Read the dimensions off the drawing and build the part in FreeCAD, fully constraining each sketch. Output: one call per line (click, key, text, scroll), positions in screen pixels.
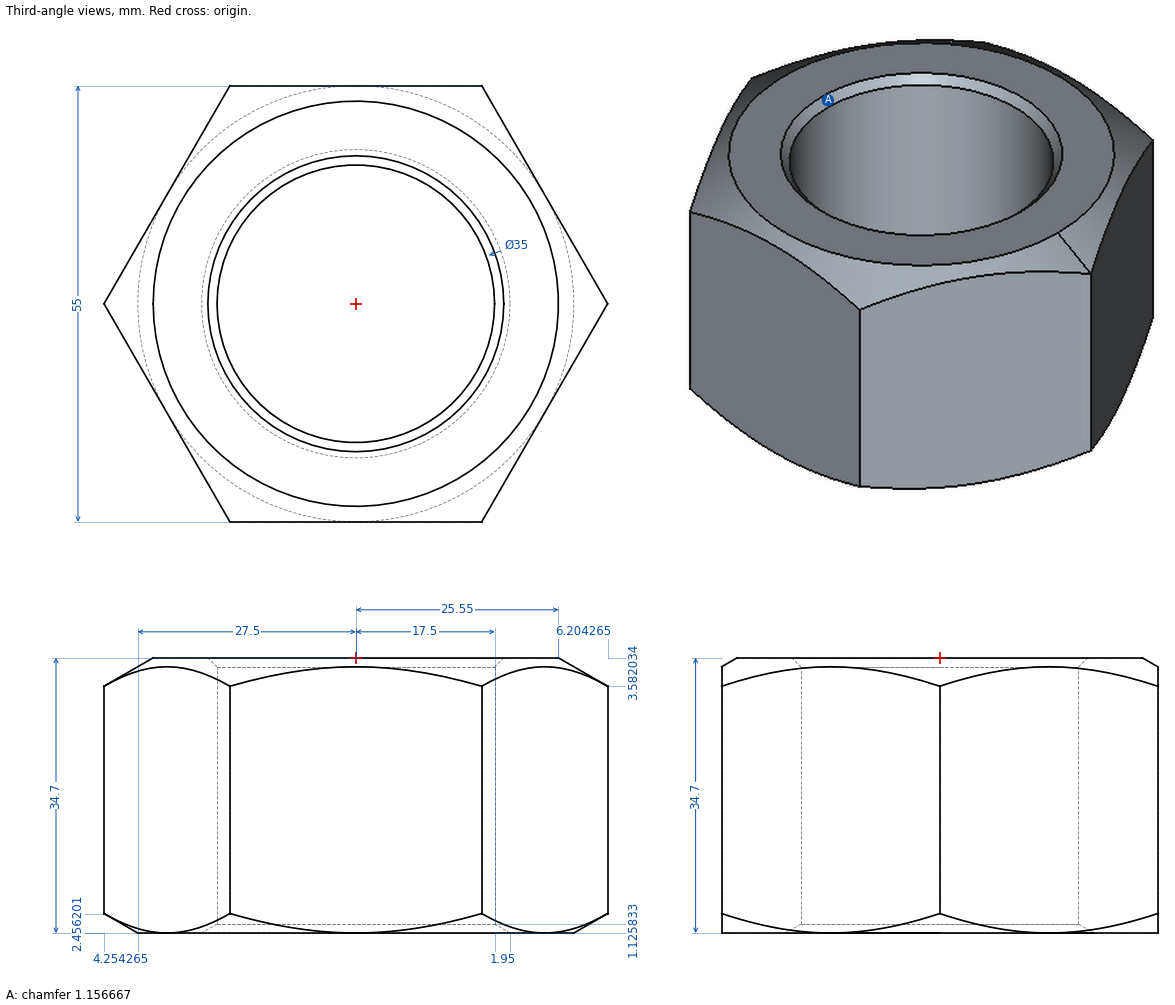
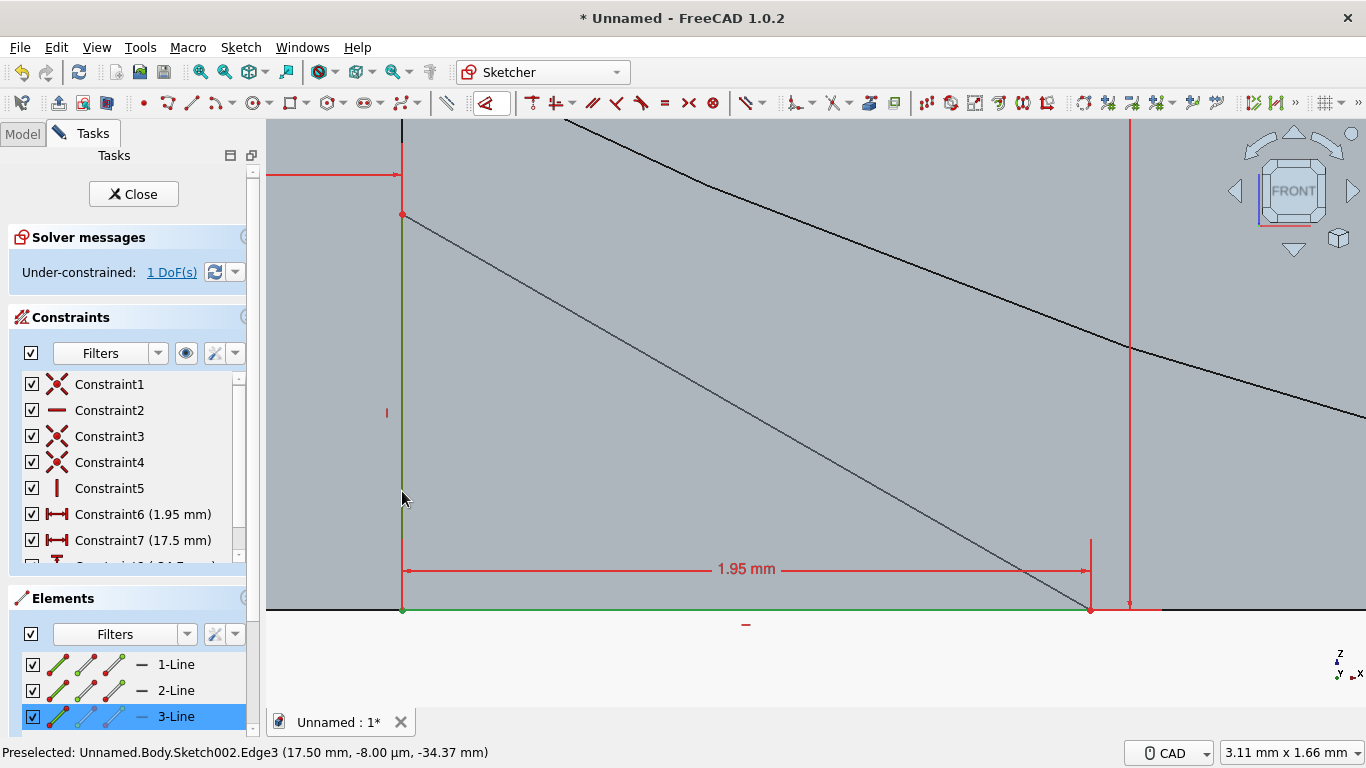
key(i)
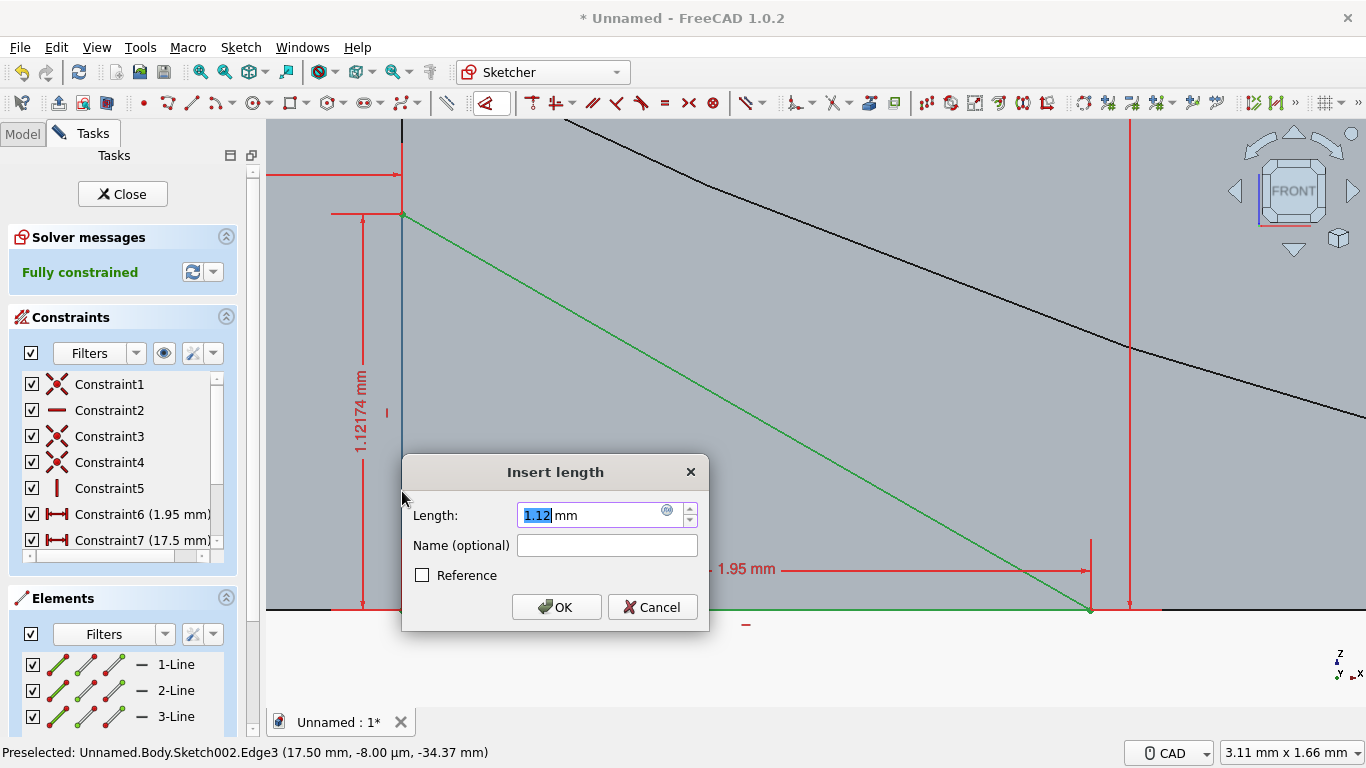
text(1.125833)
key(Return)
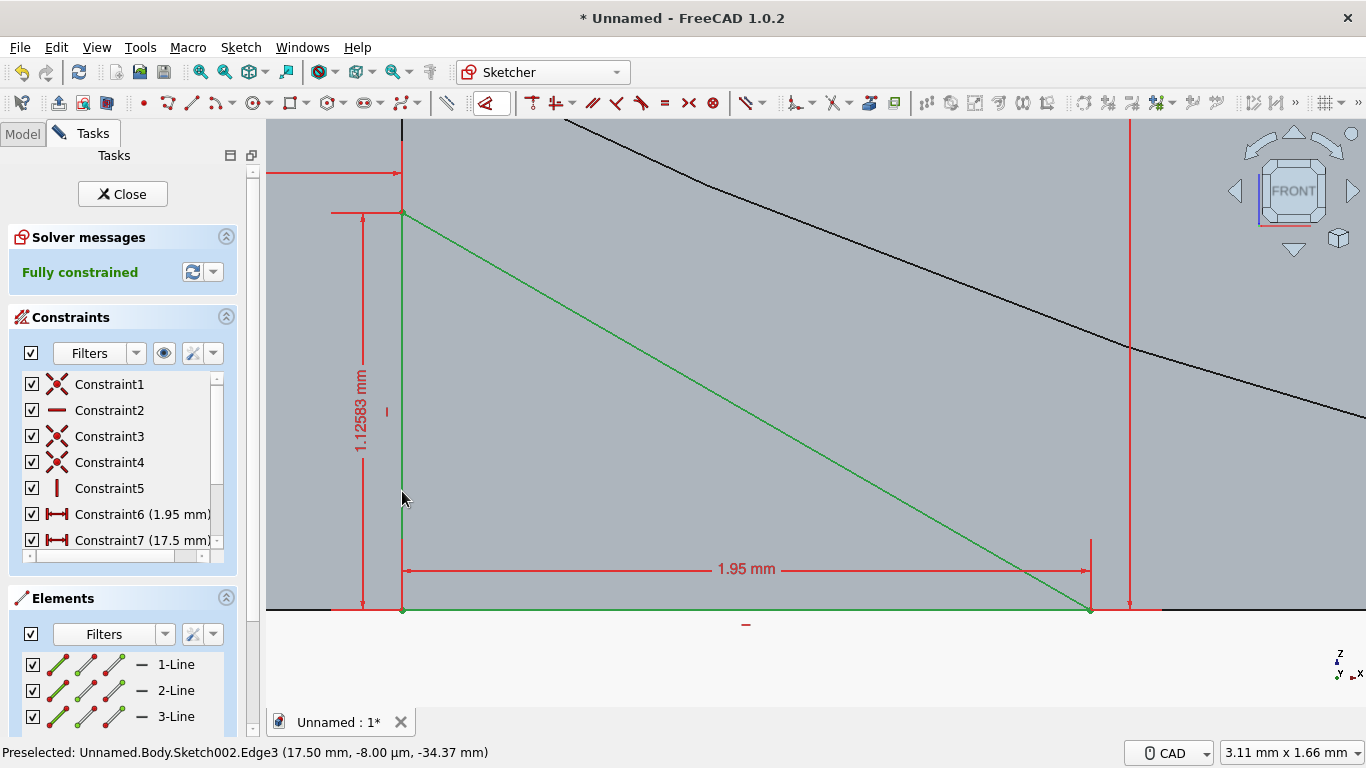
click(123, 194)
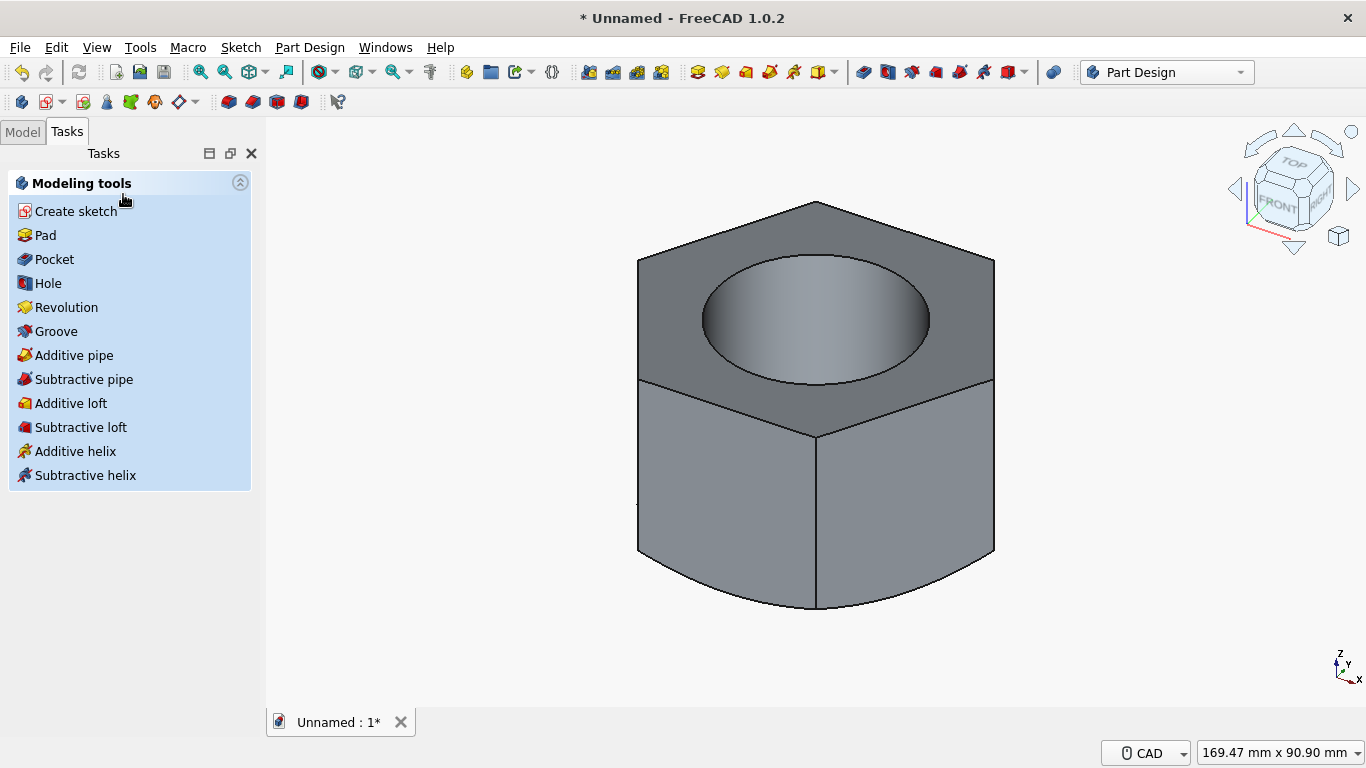
click(912, 72)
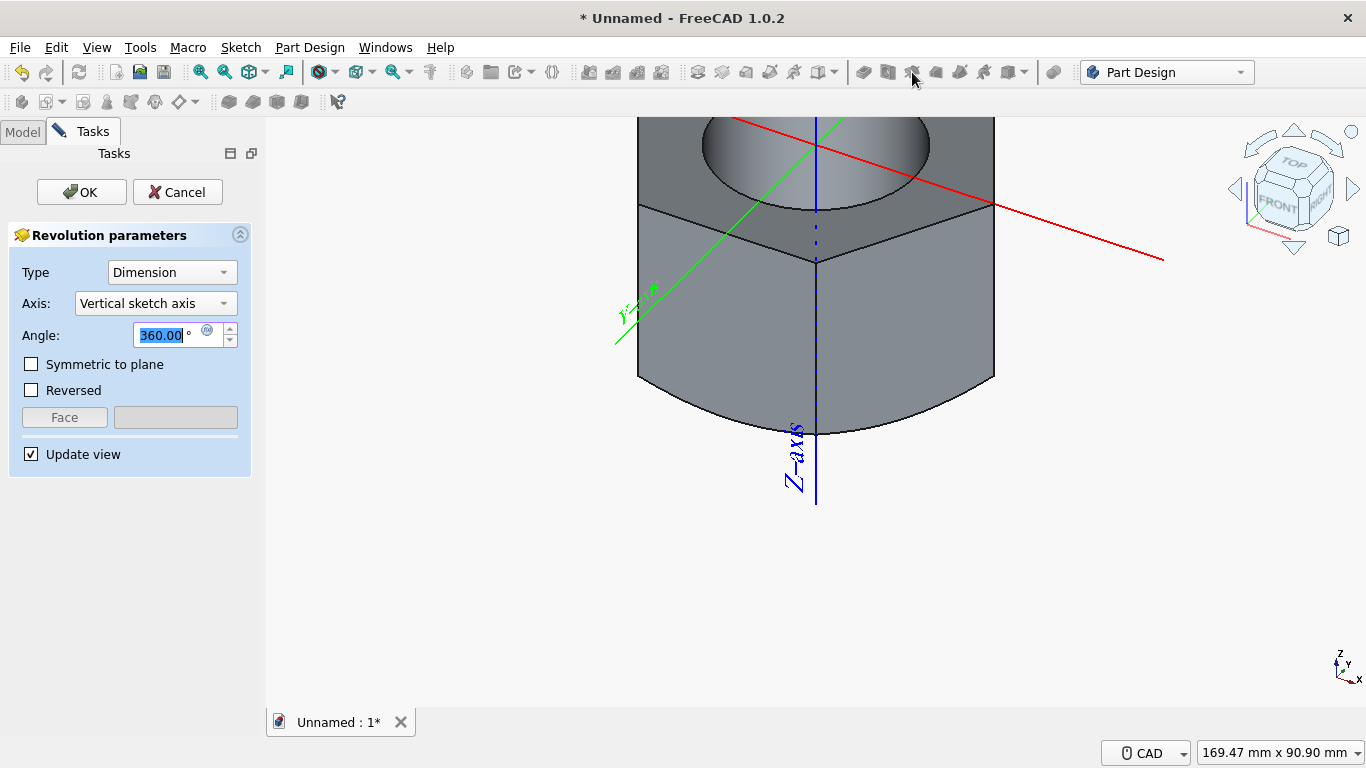
click(82, 192)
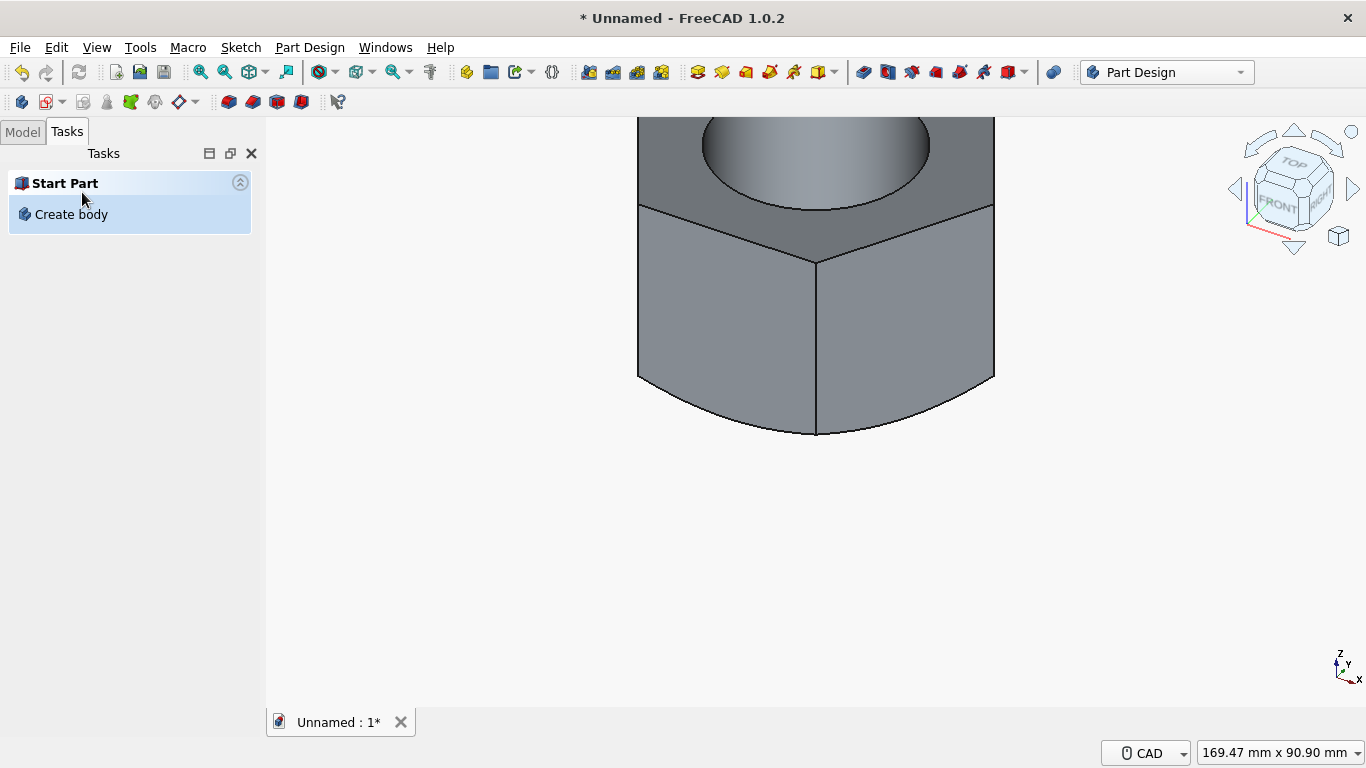
click(202, 72)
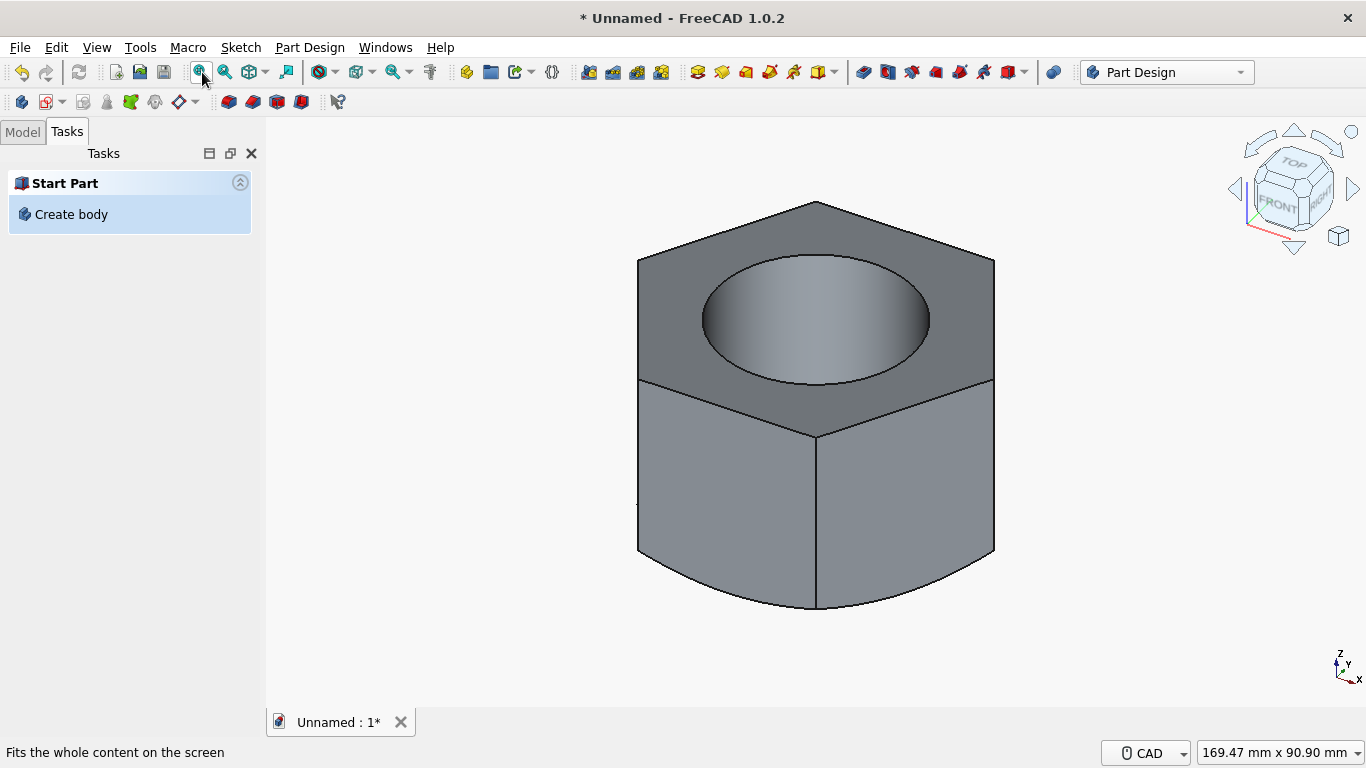
click(46, 102)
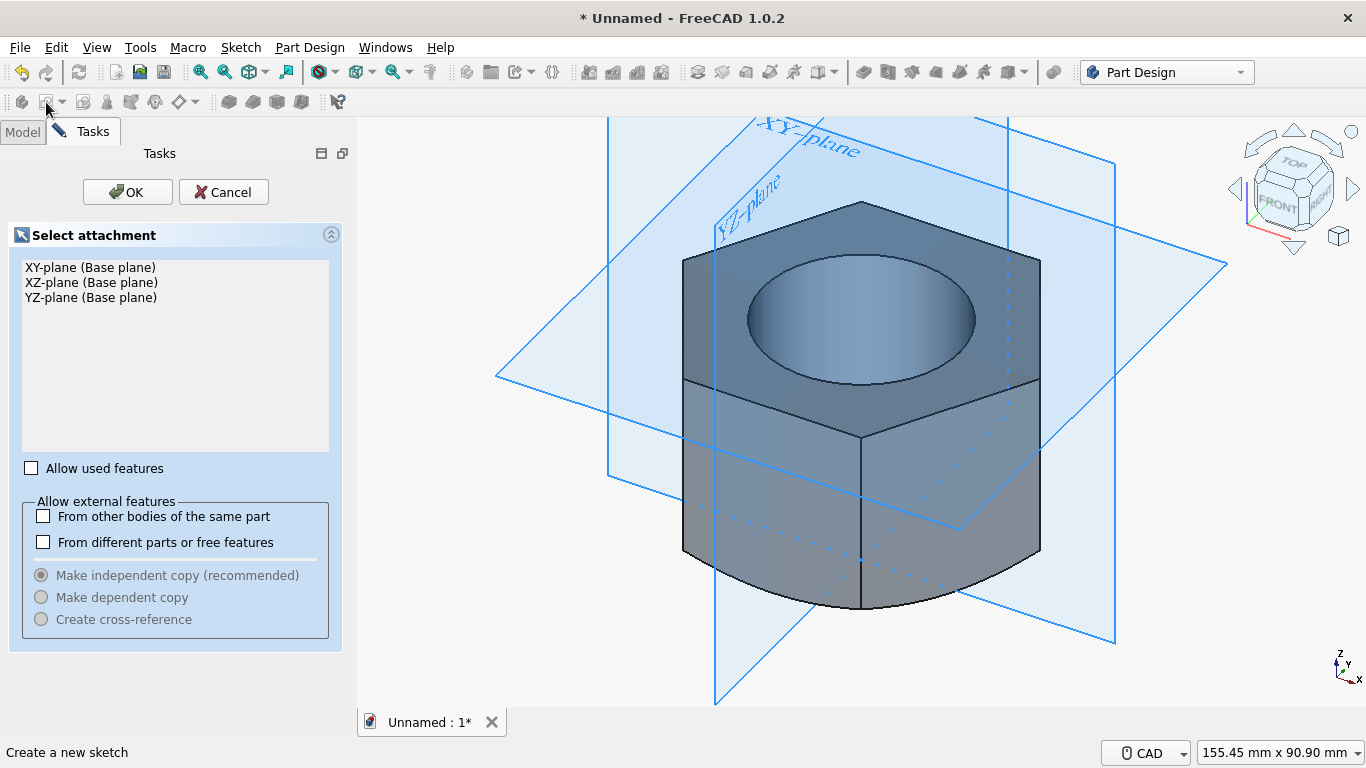
click(82, 282)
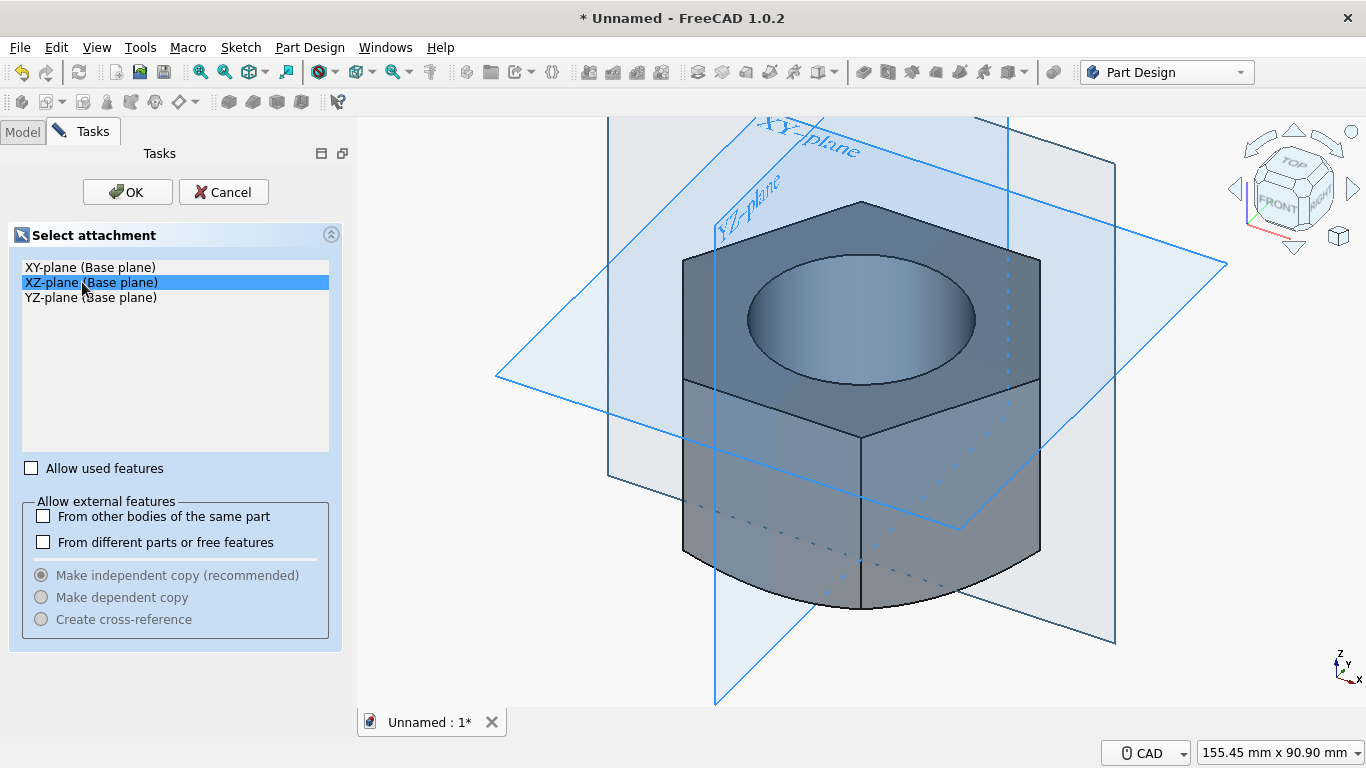
click(128, 192)